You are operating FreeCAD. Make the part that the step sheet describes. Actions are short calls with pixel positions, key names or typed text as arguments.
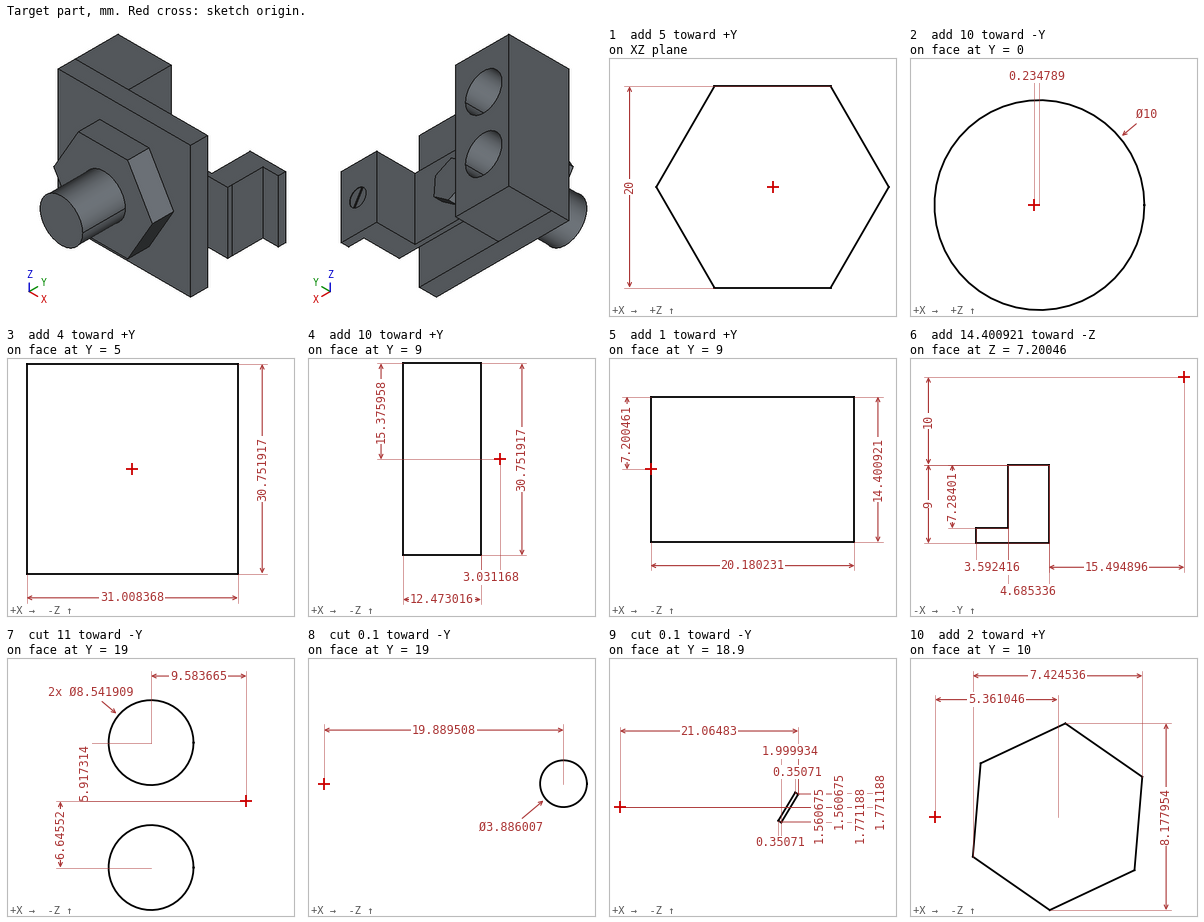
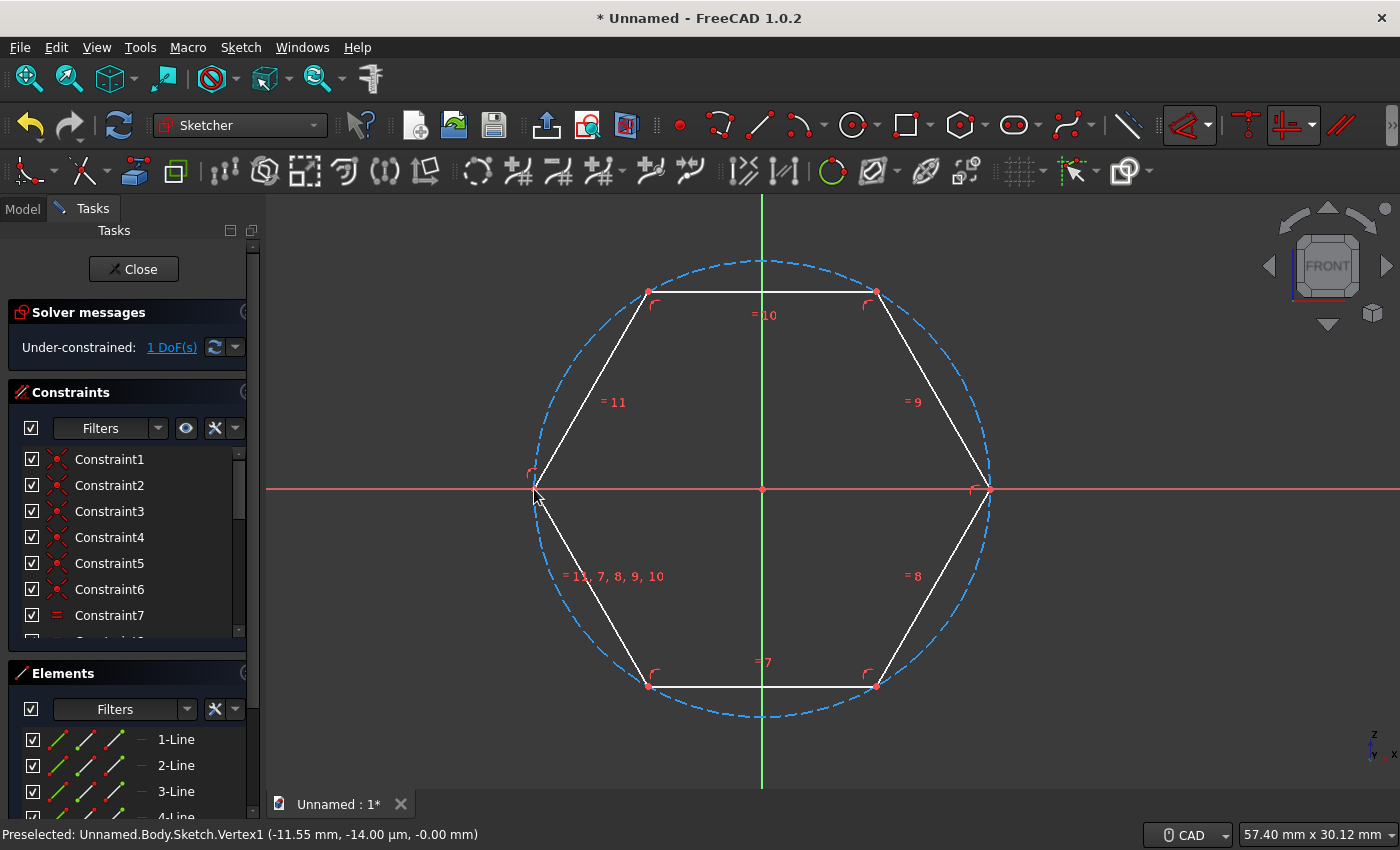
click(1184, 126)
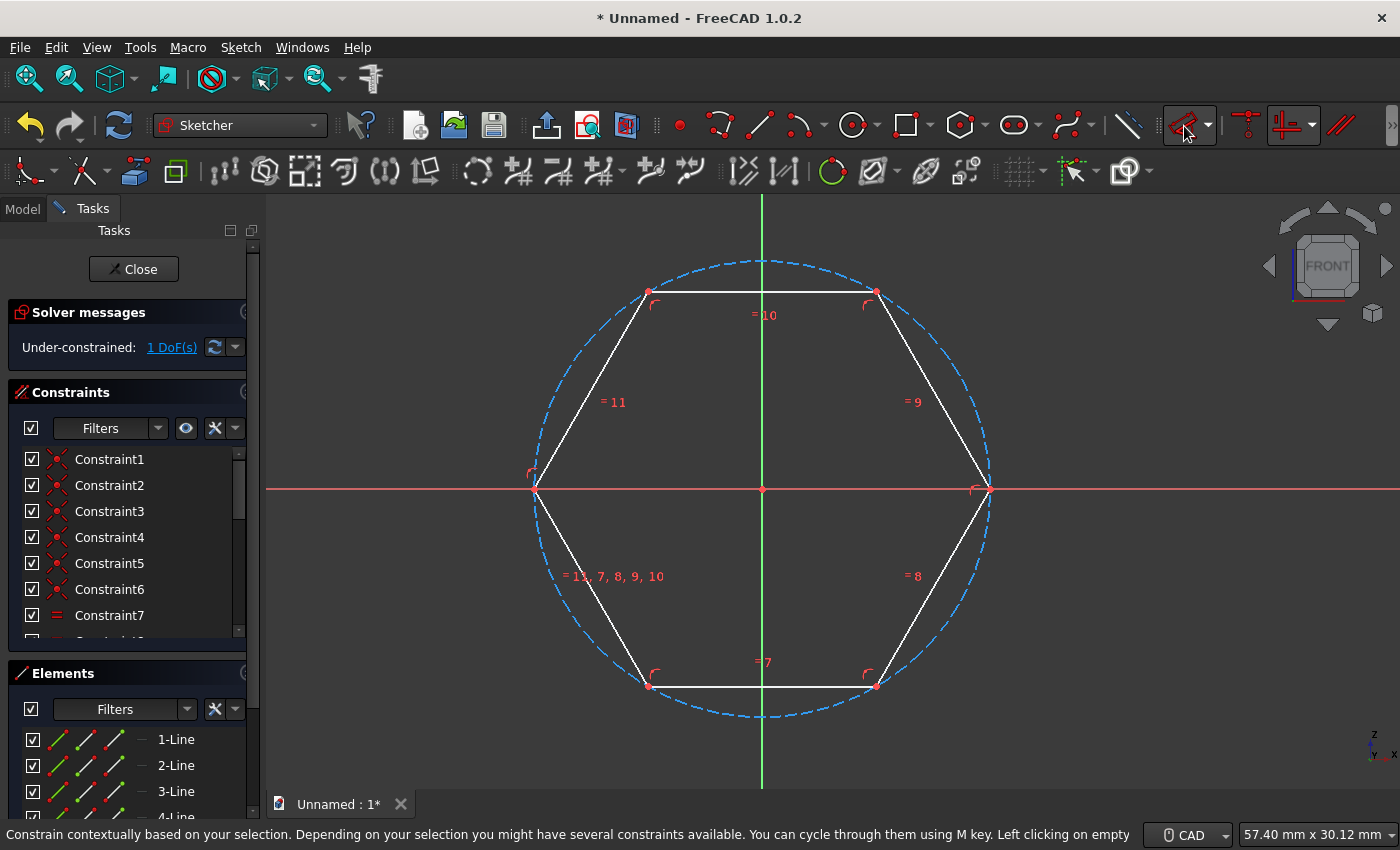
click(648, 687)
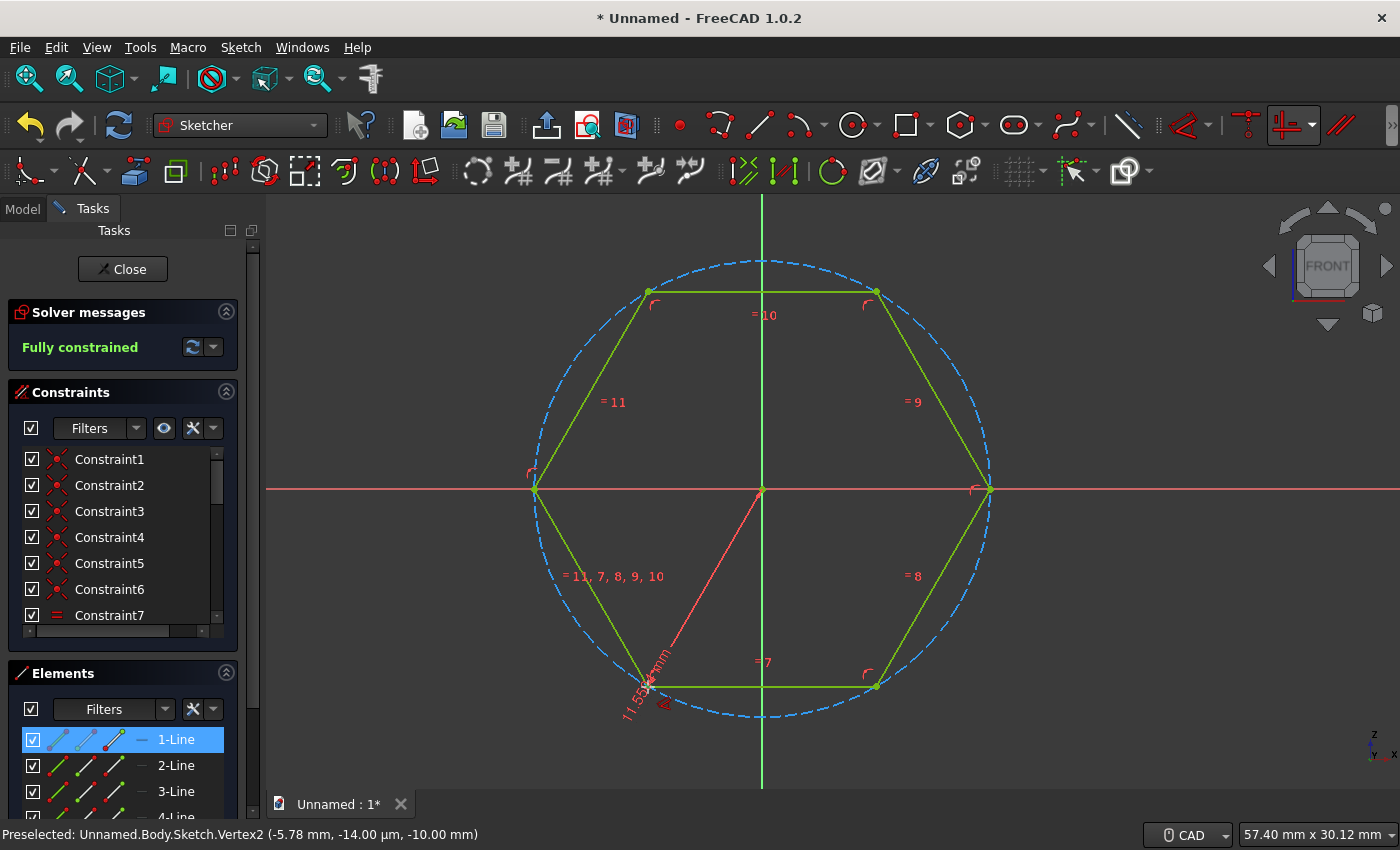
click(876, 292)
click(910, 398)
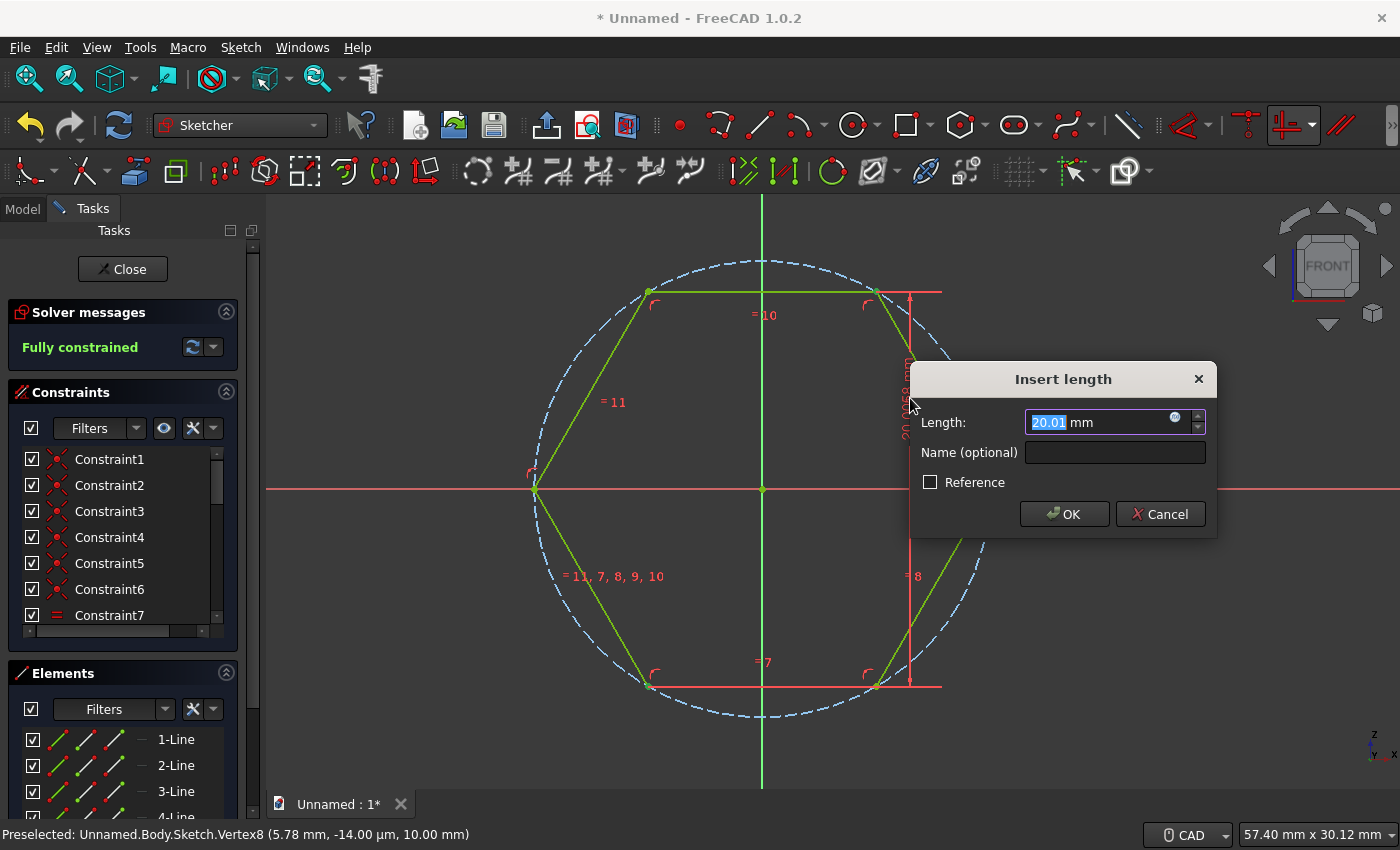
text(20)
key(Return)
key(Escape)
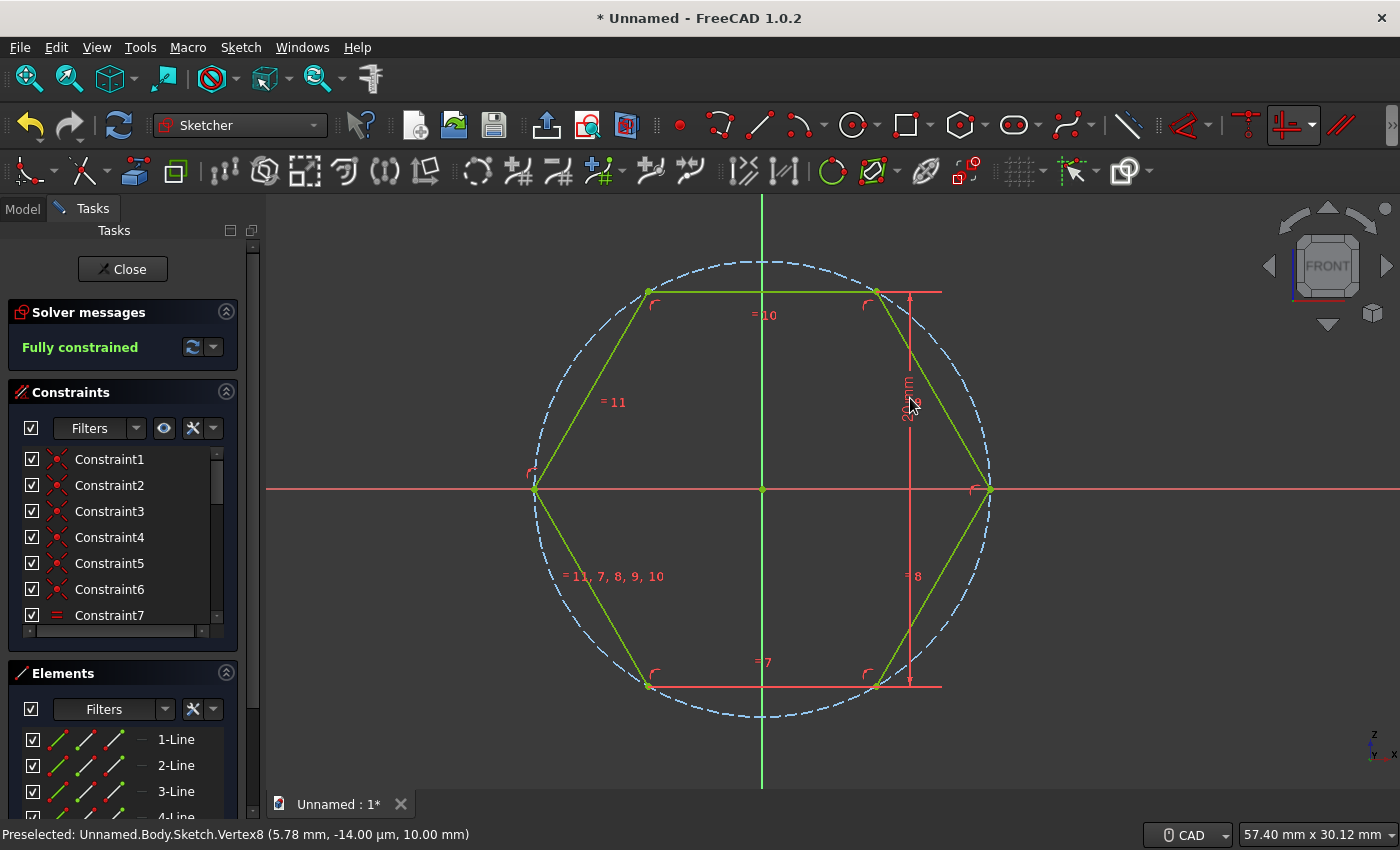
click(123, 269)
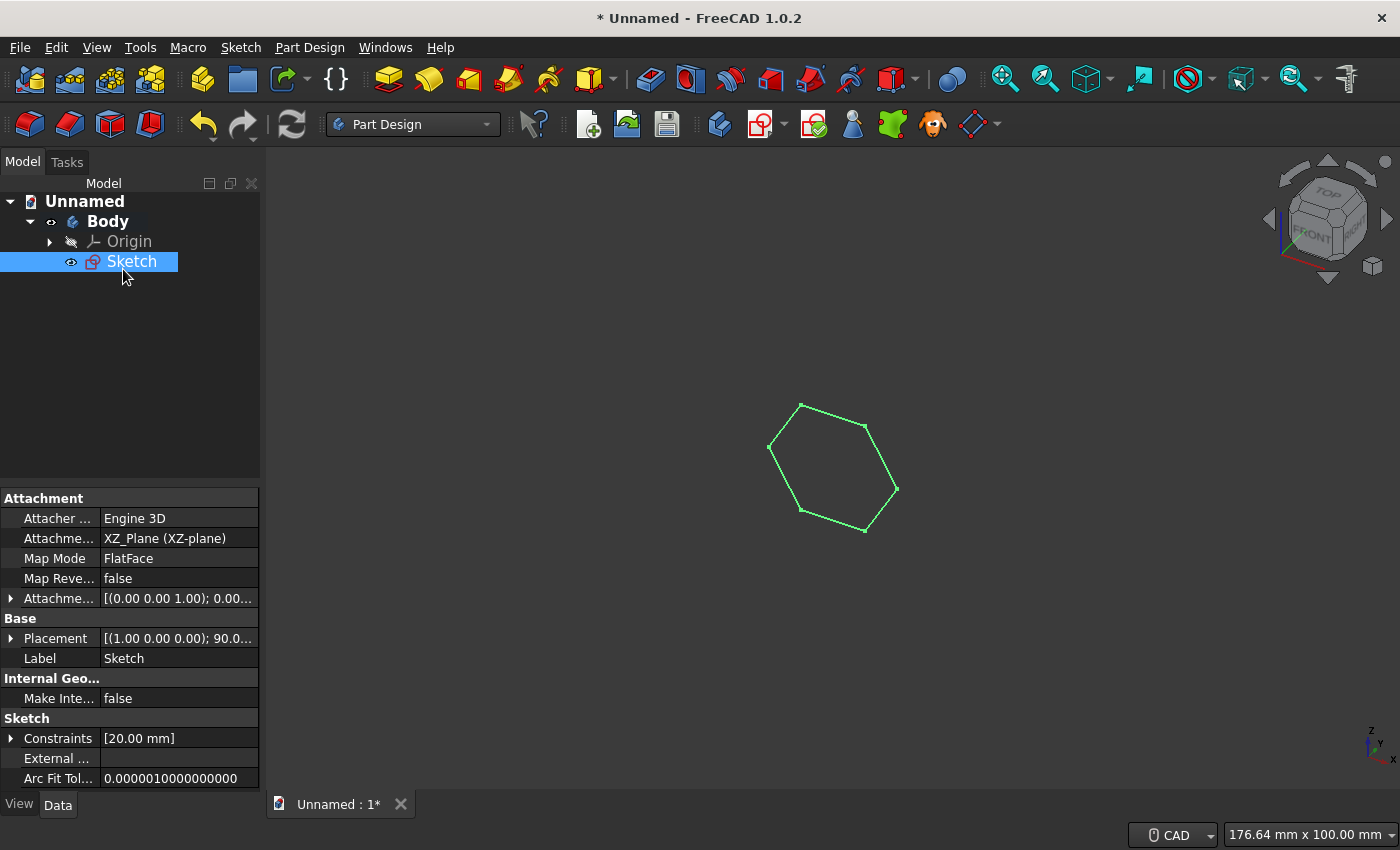
click(390, 80)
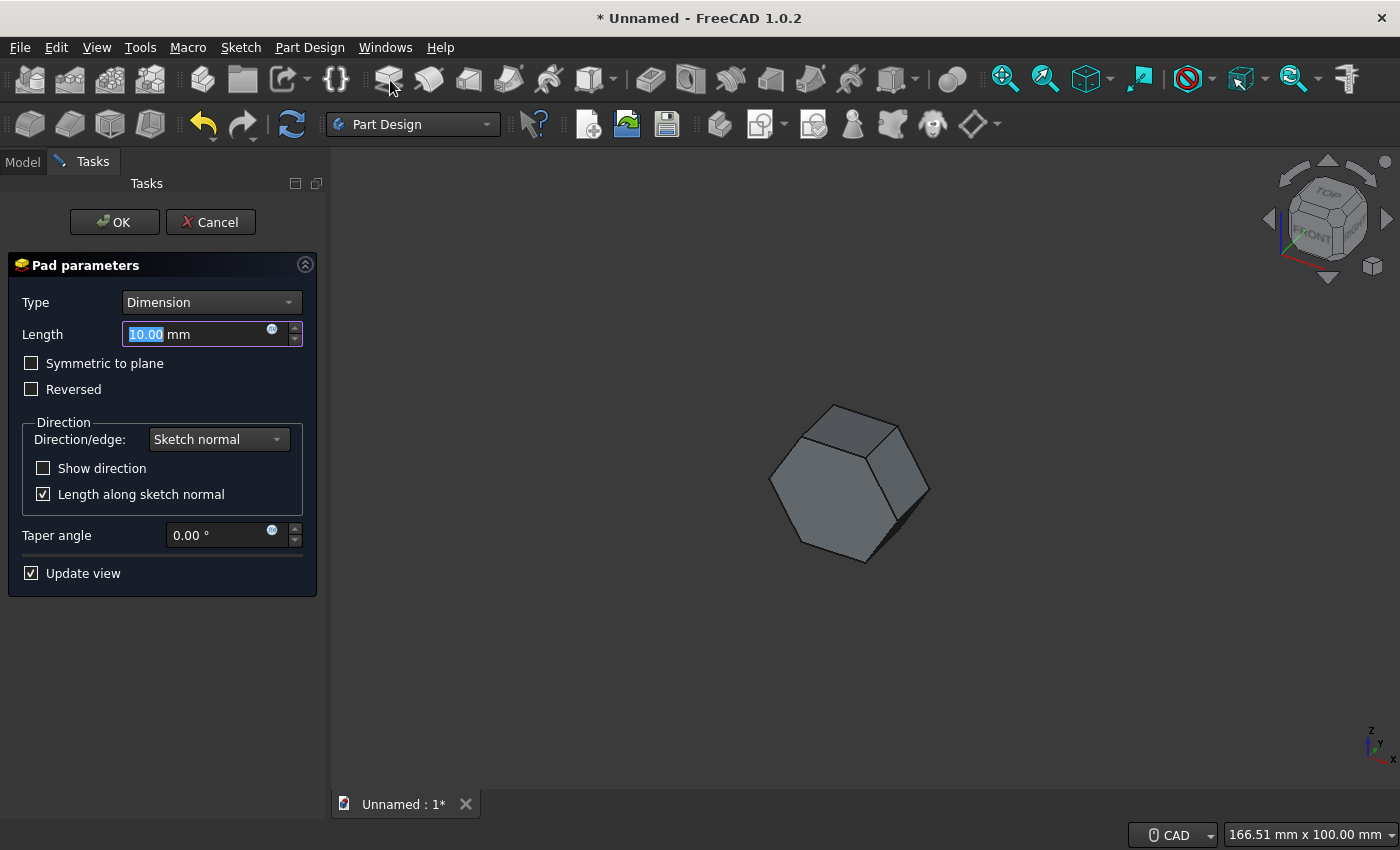
text(5)
key(Tab)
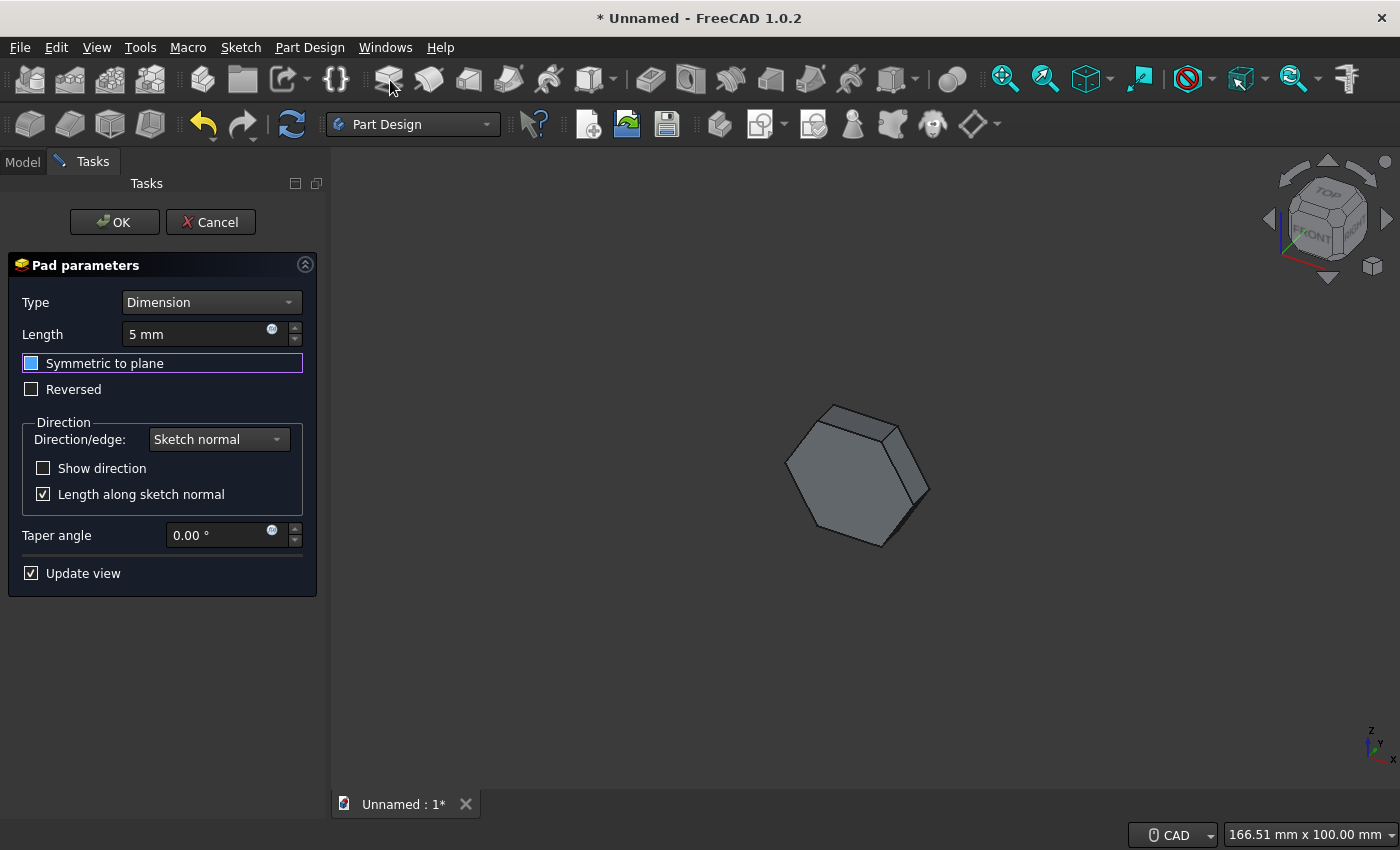
click(30, 389)